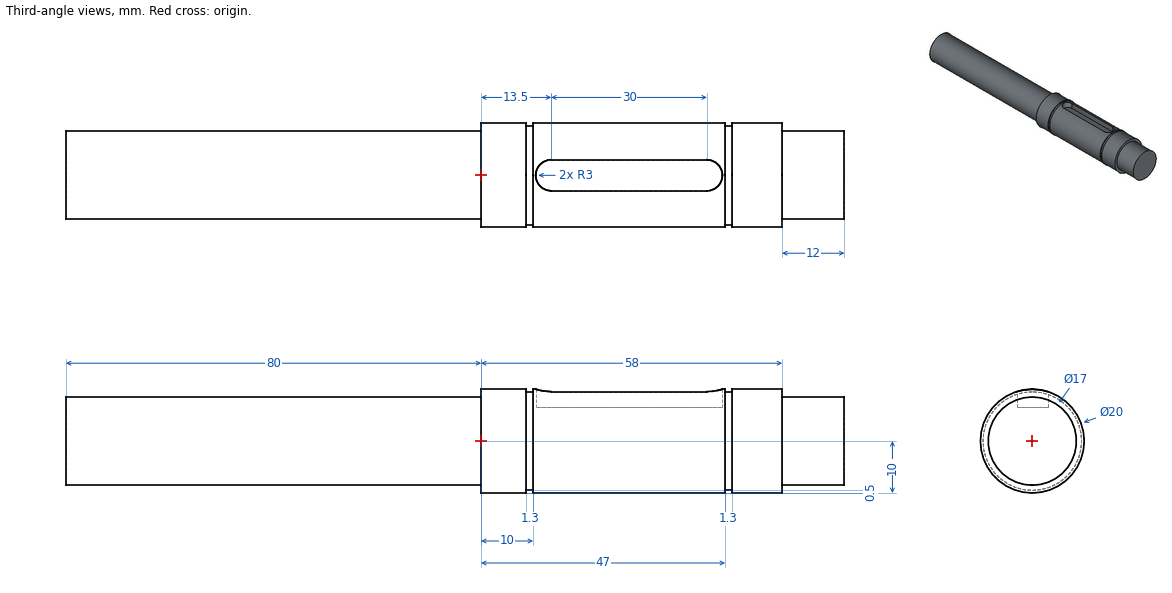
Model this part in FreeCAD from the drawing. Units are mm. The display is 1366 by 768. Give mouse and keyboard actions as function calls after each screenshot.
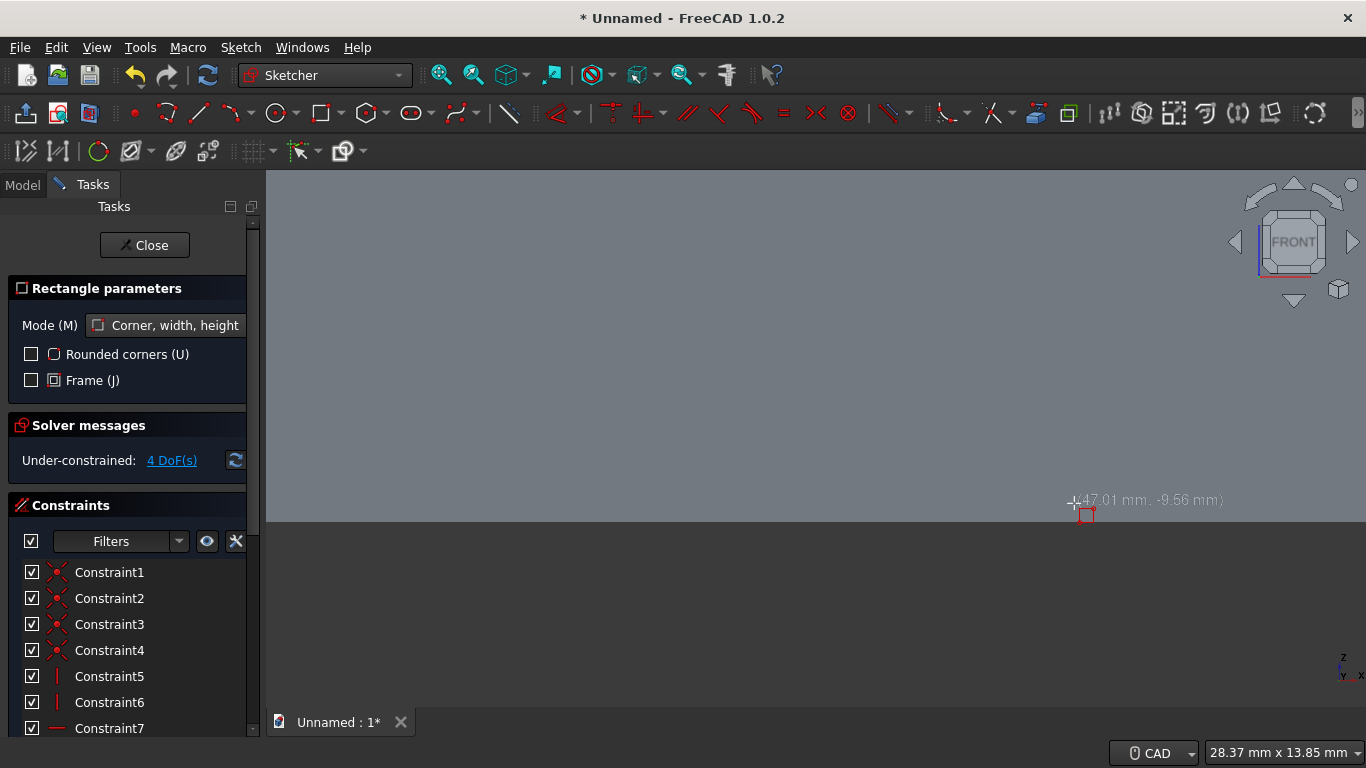
click(1072, 502)
click(1123, 522)
key(Escape)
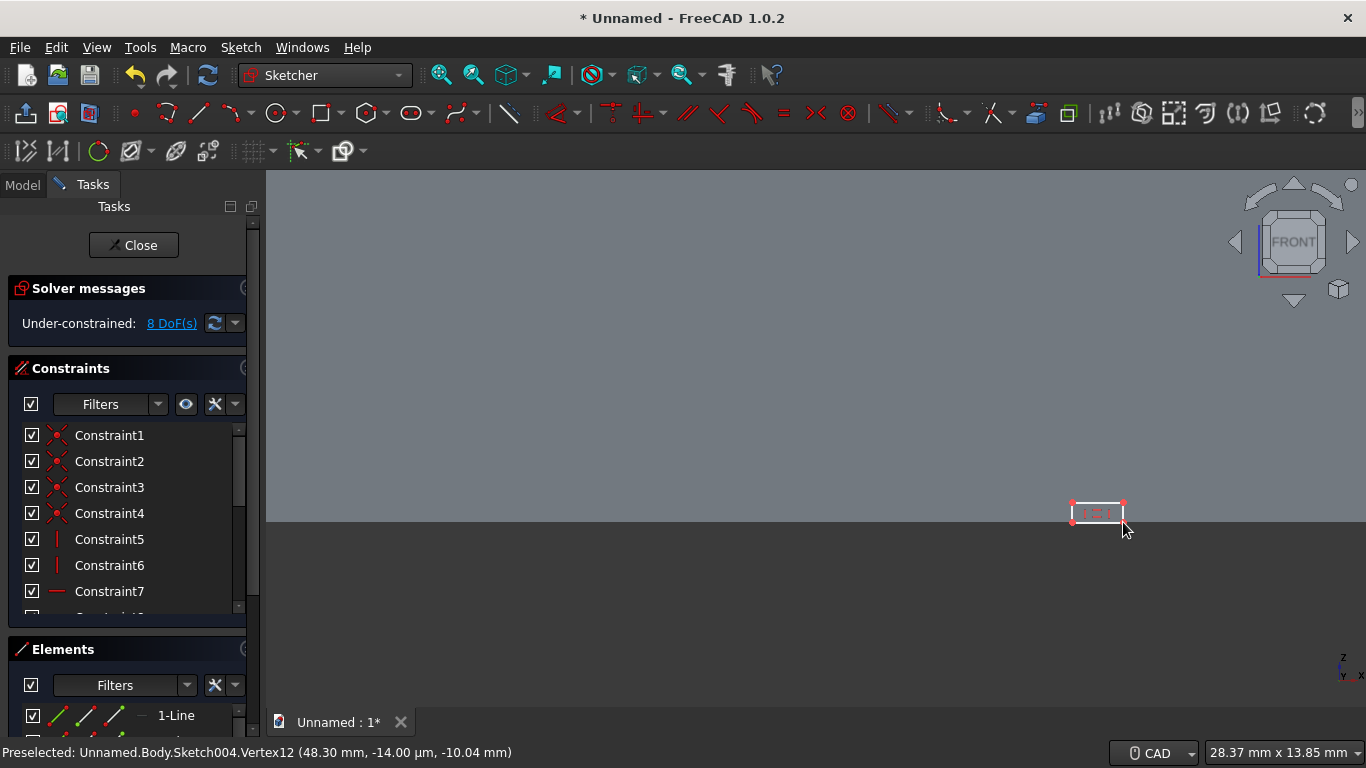
key(d)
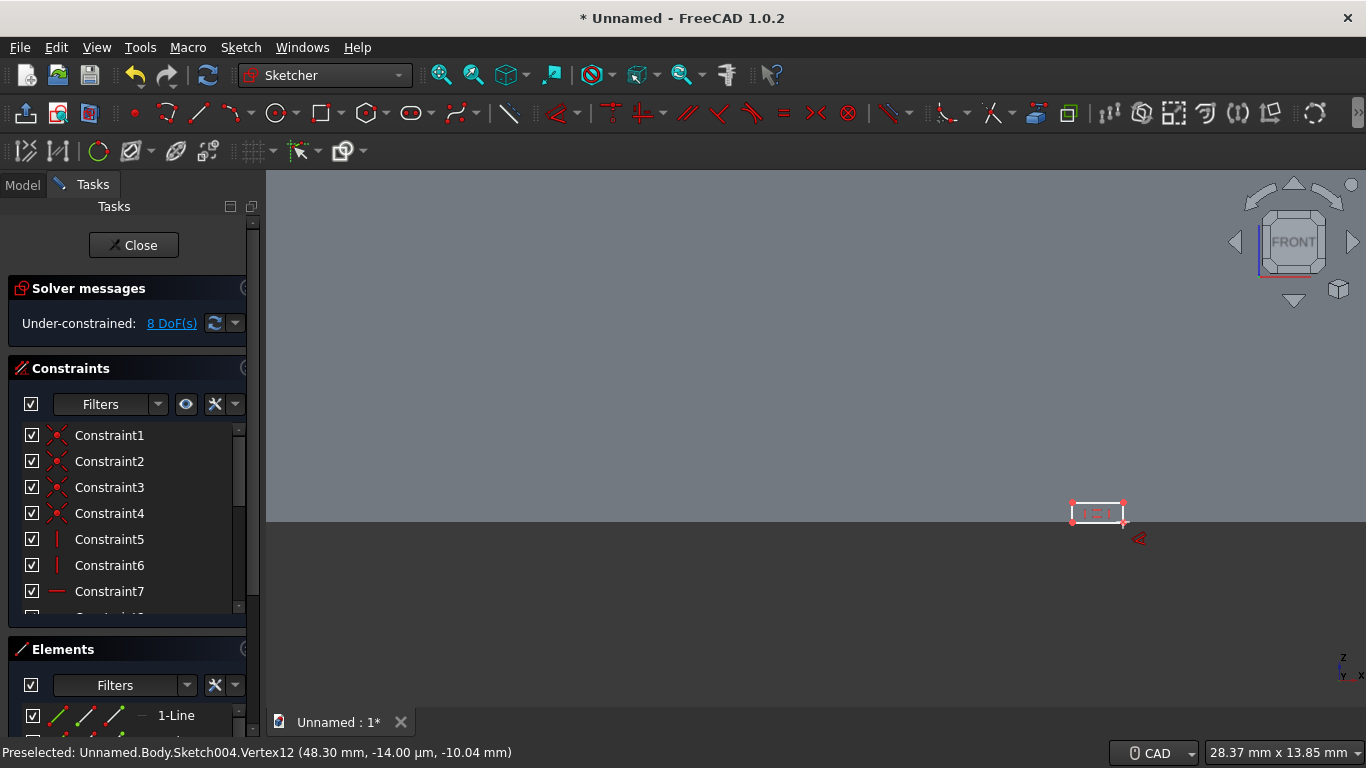
scroll(1074, 503, down, 5)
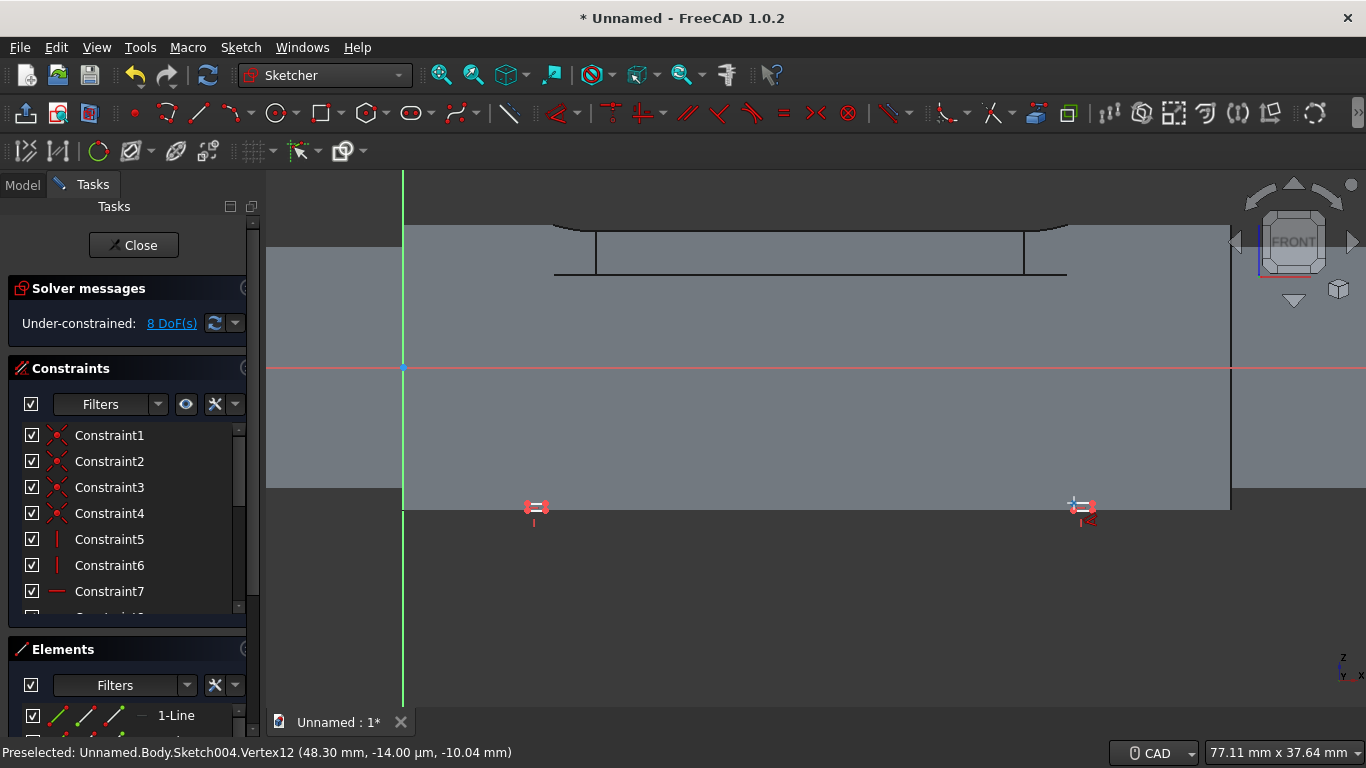
scroll(528, 507, up, 9)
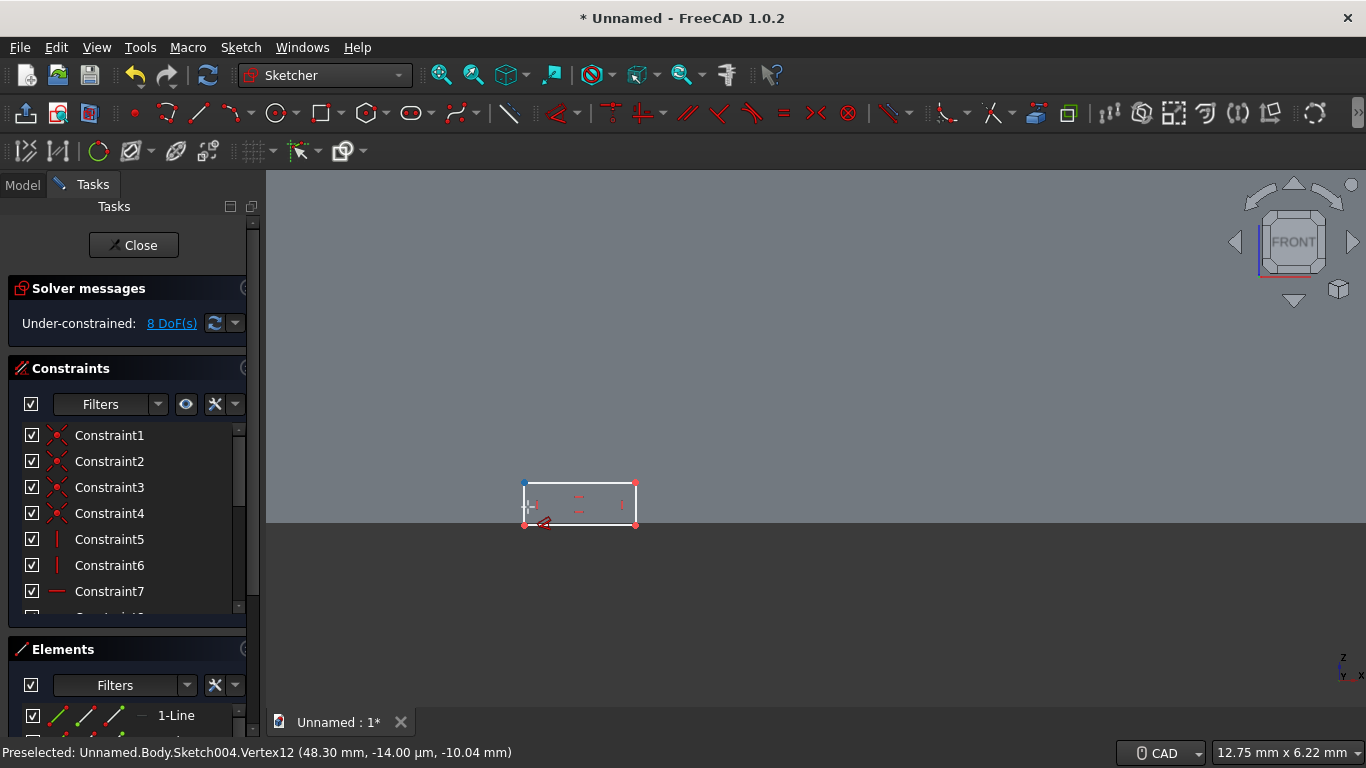
click(524, 504)
click(490, 504)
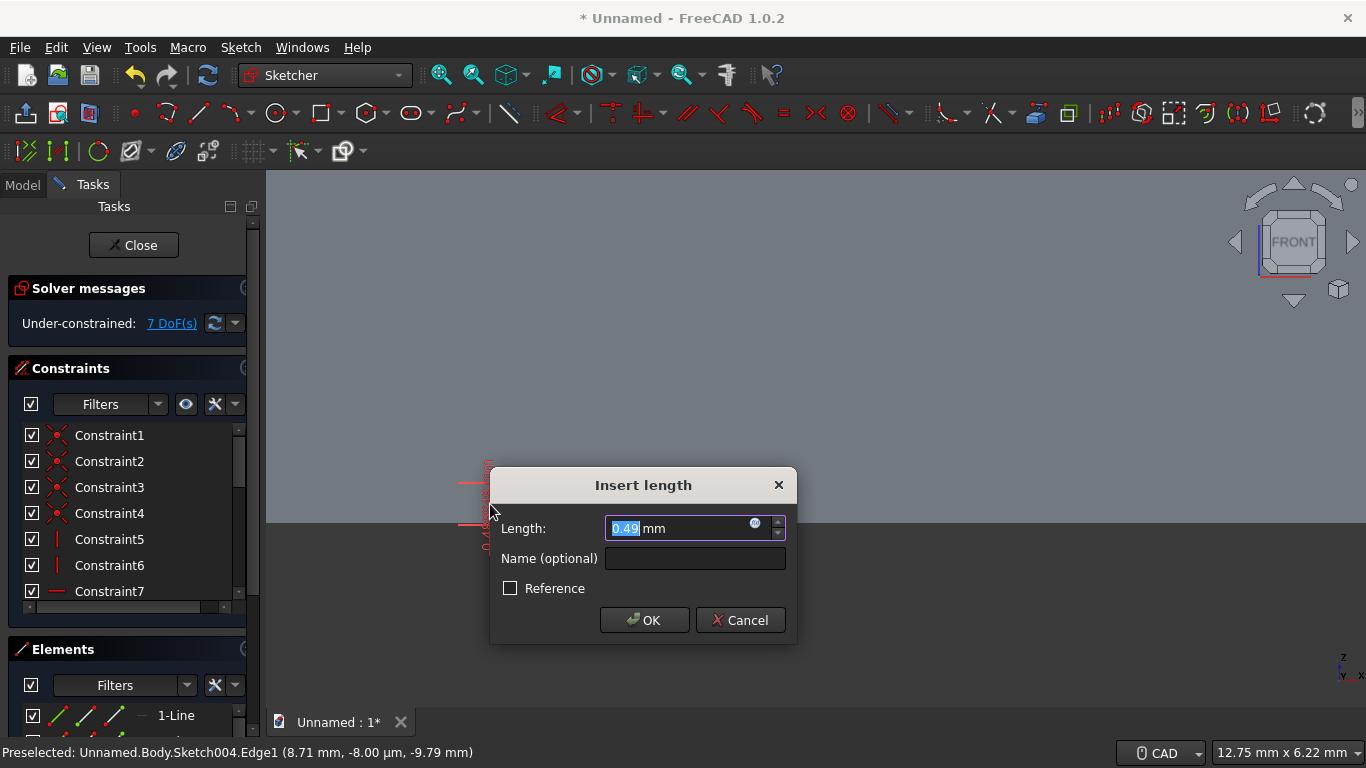
text(0.5)
key(Return)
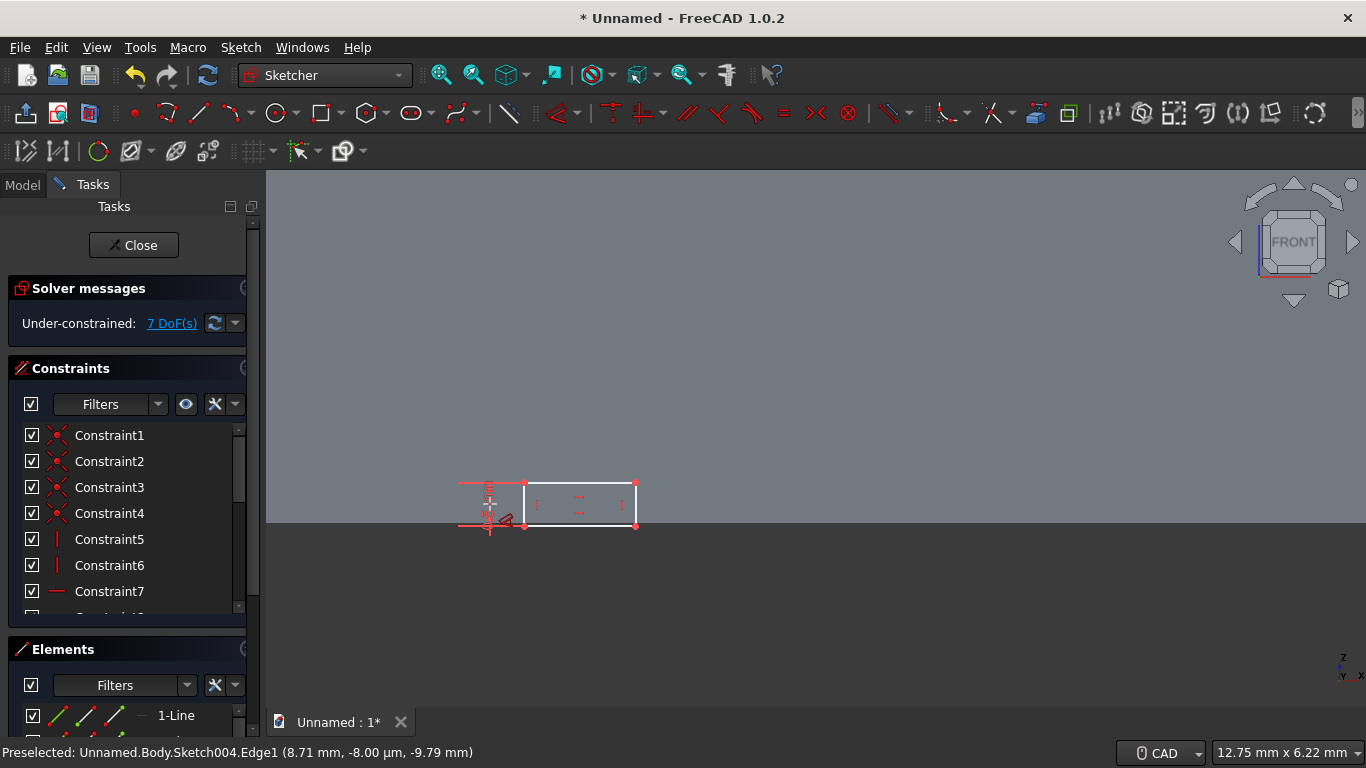
click(558, 526)
click(580, 560)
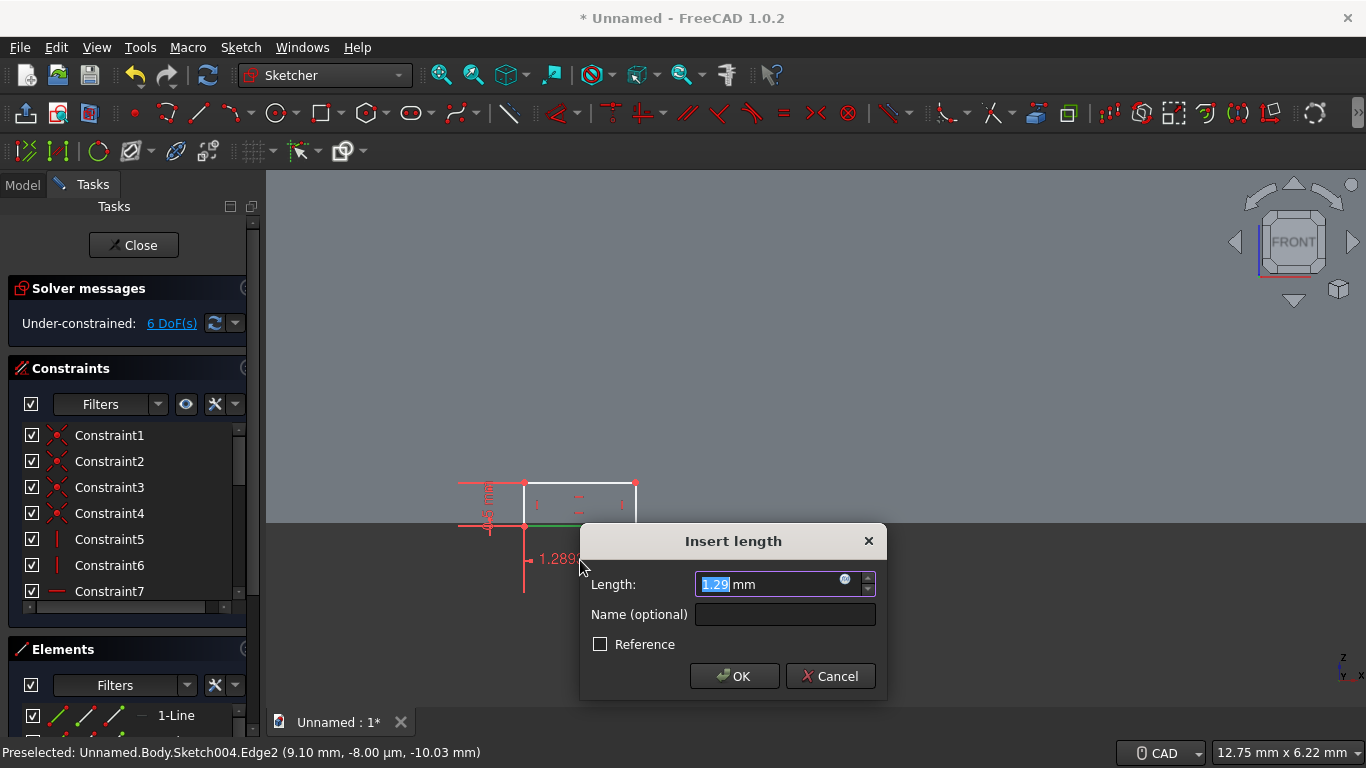
text(1.3)
key(Return)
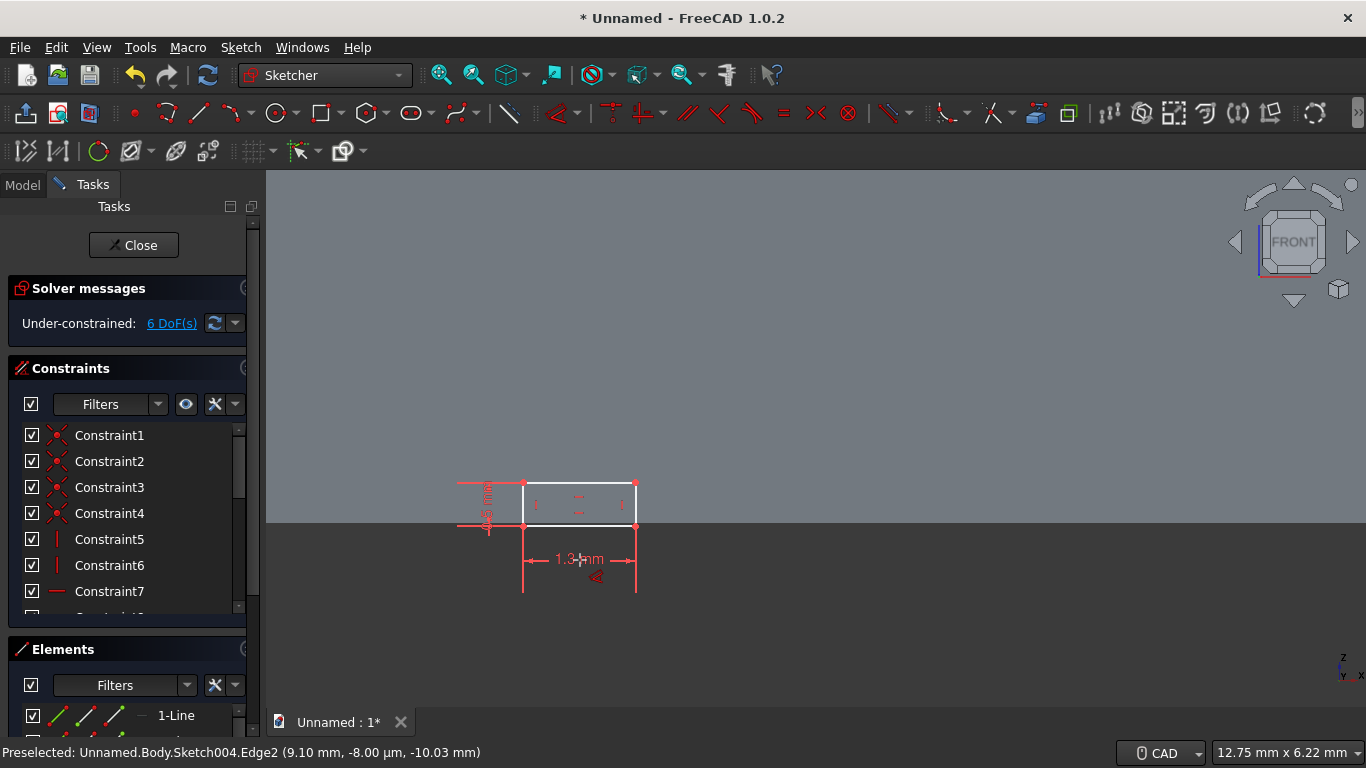
scroll(528, 507, down, 9)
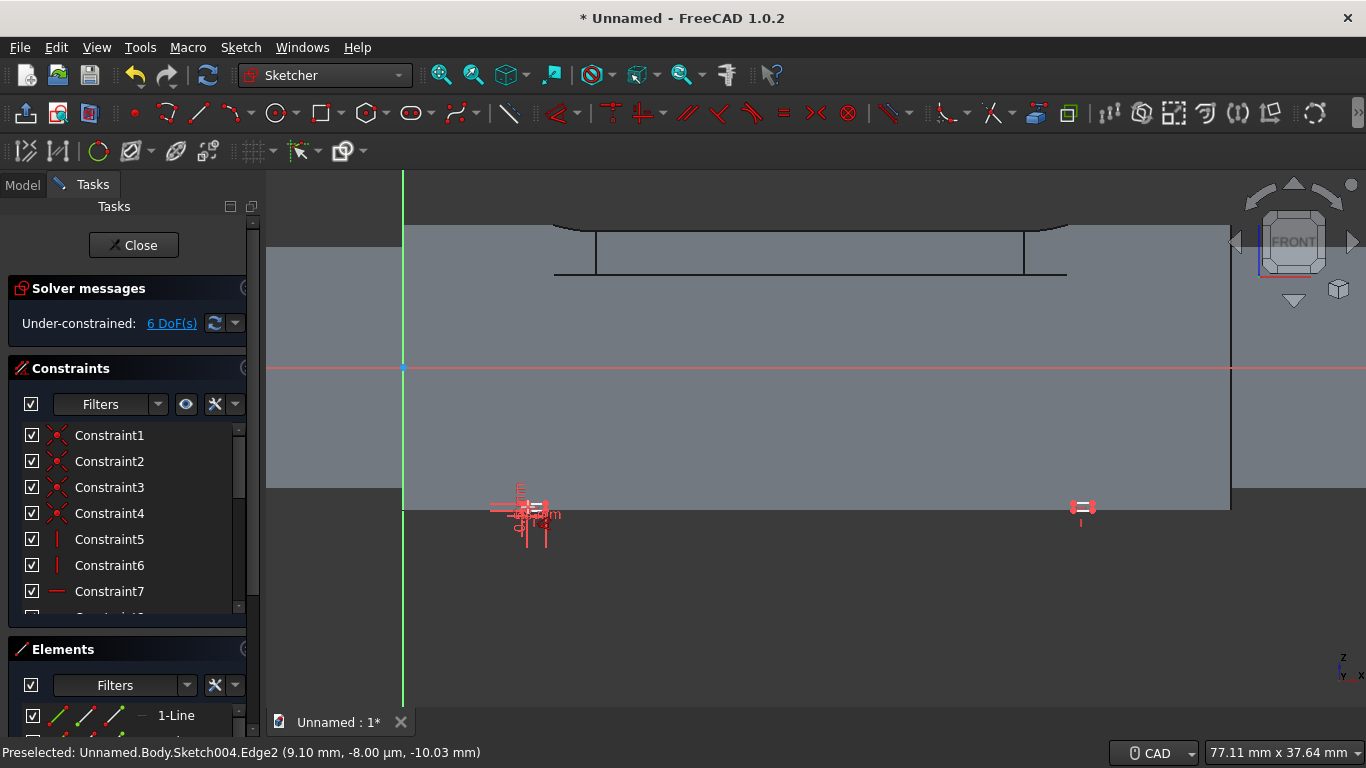
scroll(1074, 506, up, 10)